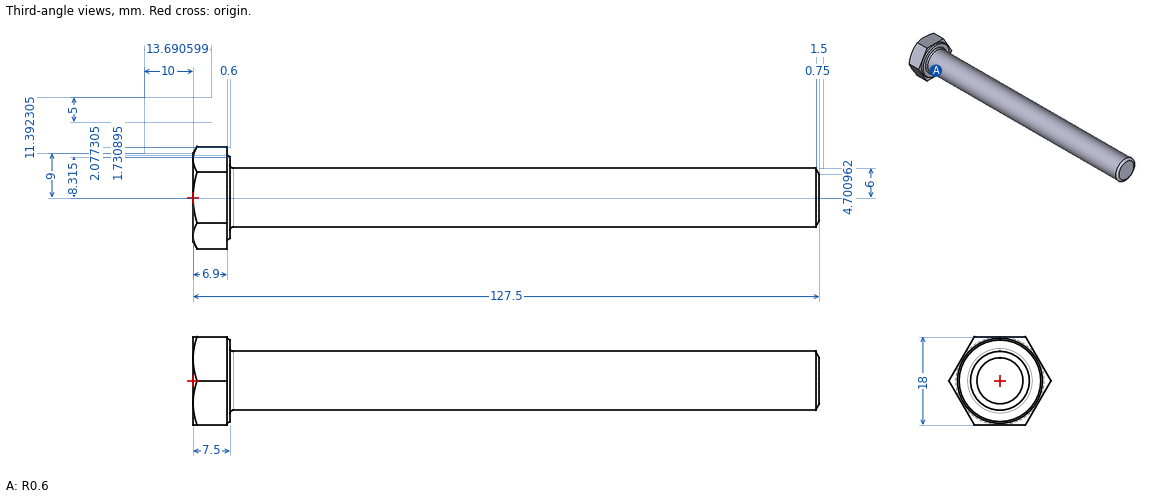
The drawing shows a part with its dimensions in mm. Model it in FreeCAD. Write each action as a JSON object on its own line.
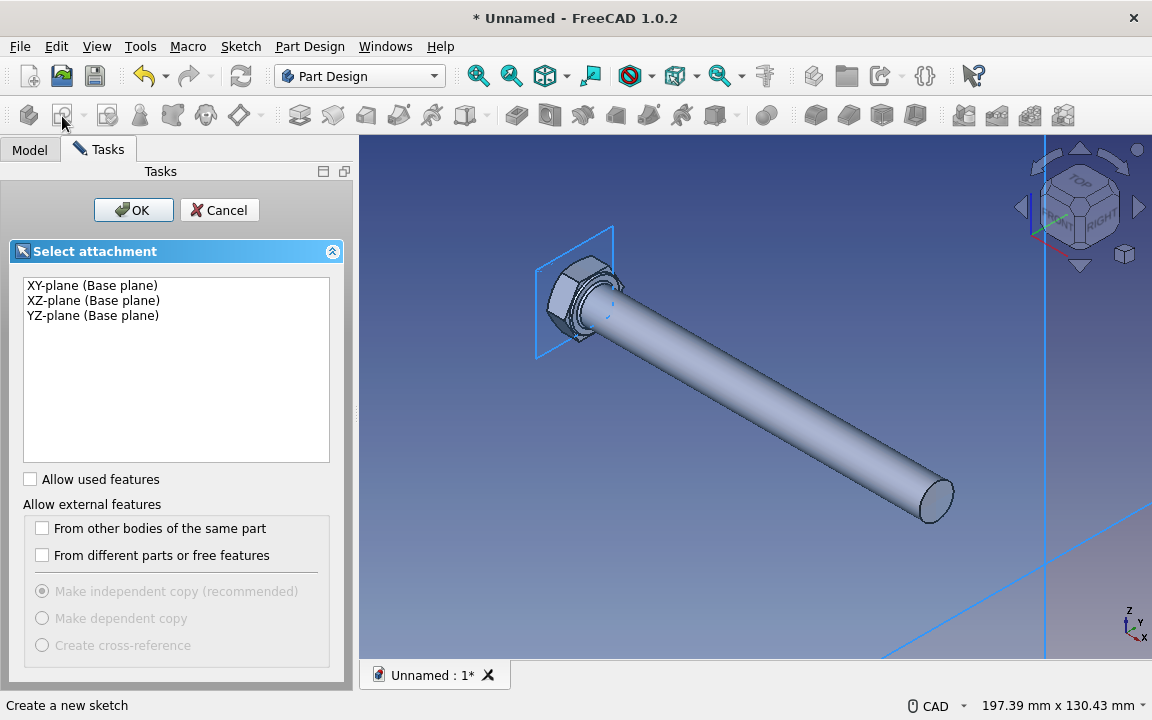
{"action": "left_click", "coordinate": [84, 286]}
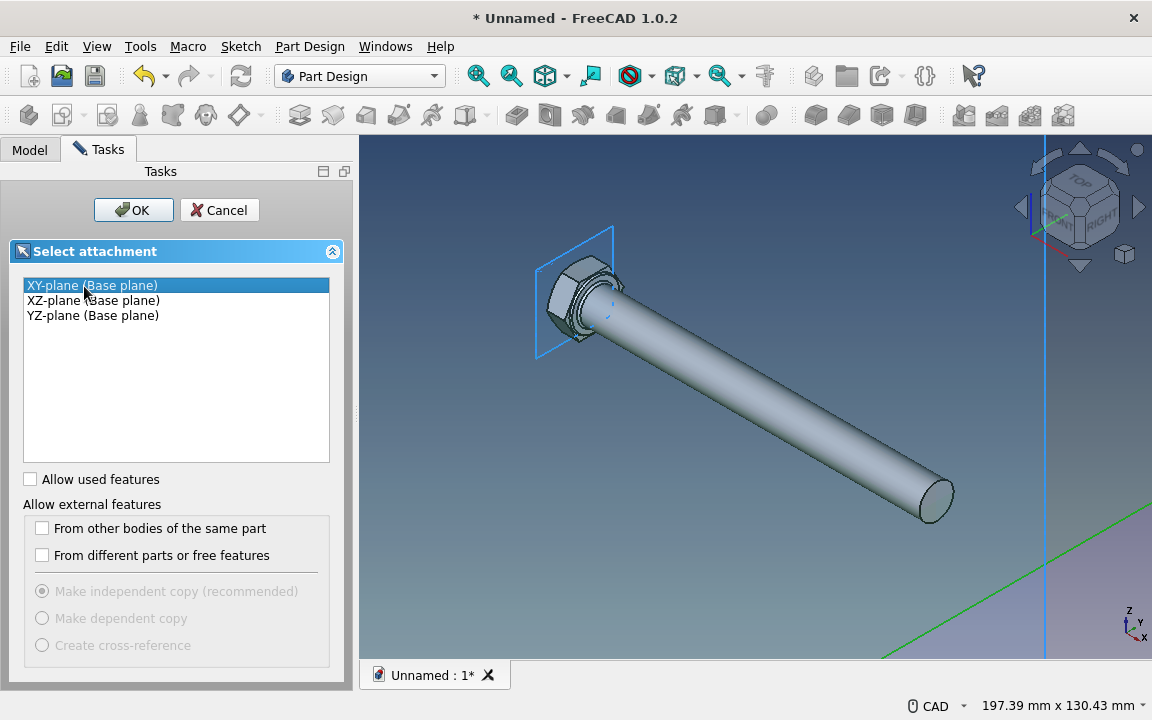
{"action": "left_click", "coordinate": [134, 210]}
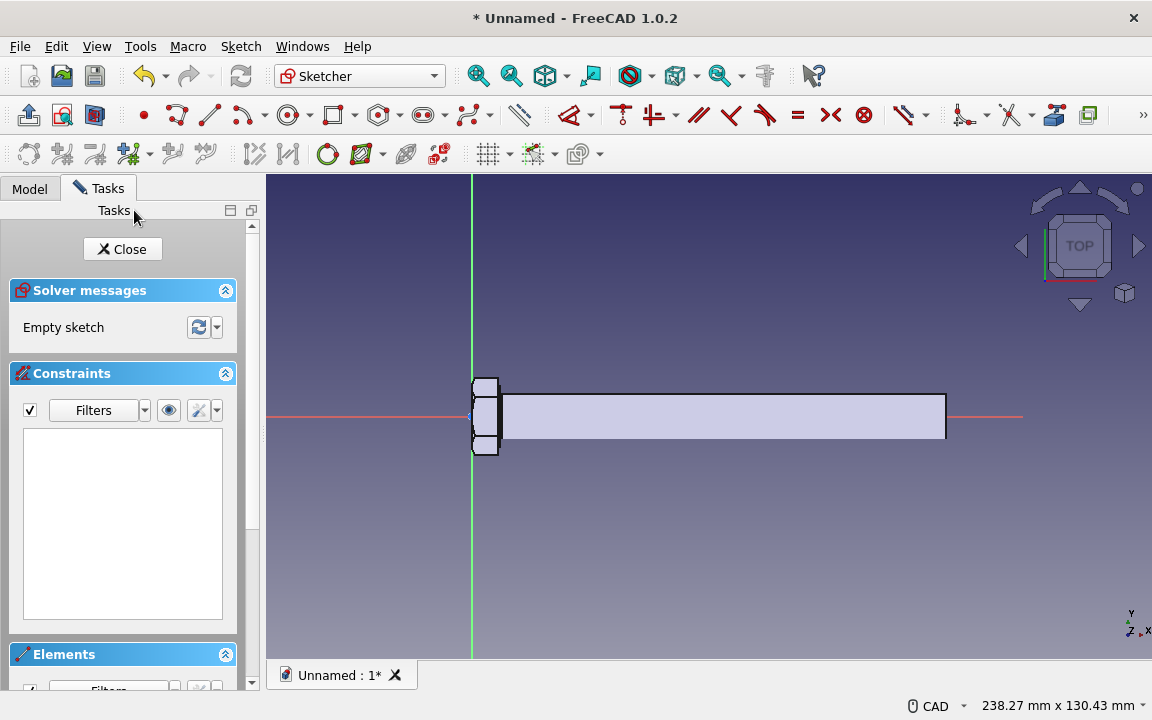
{"action": "left_click", "coordinate": [95, 116]}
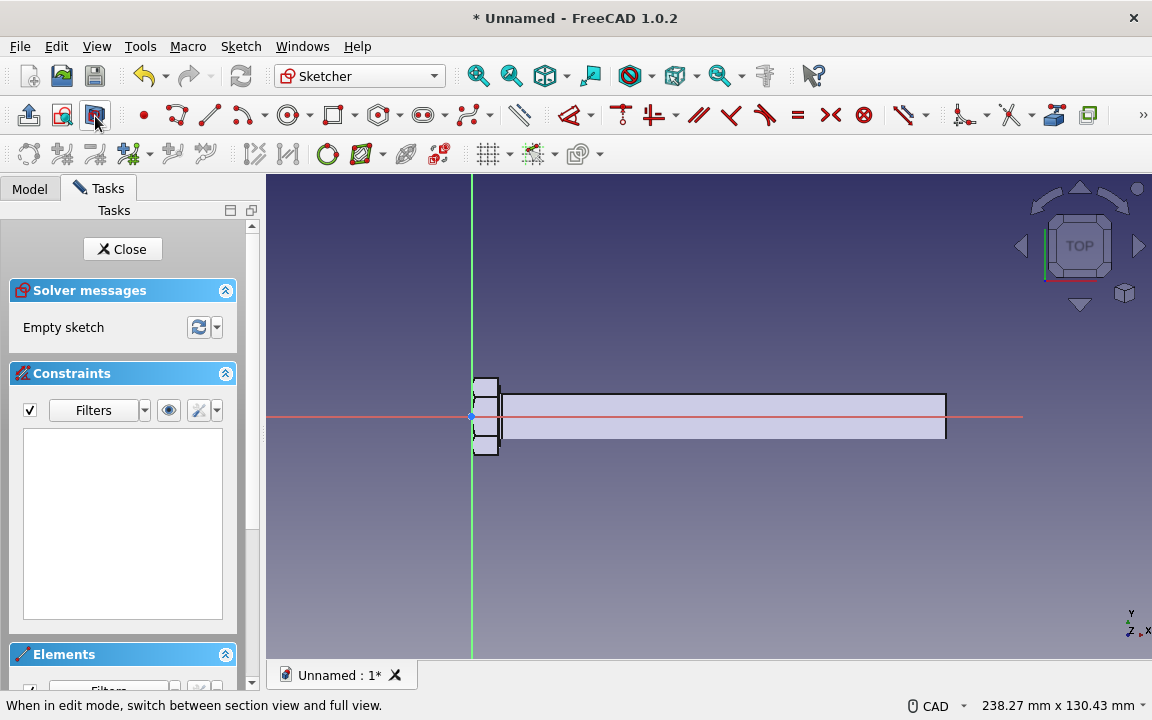
{"action": "scroll", "coordinate": [962, 396], "scroll_direction": "up", "scroll_amount": 15}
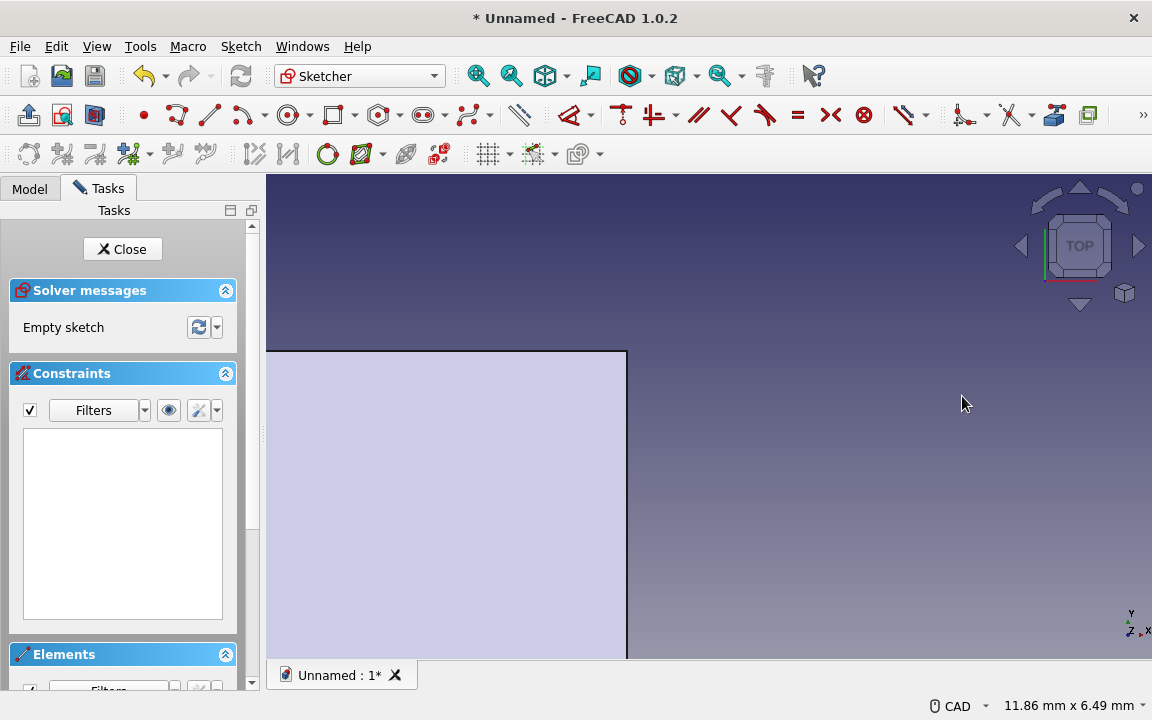
{"action": "scroll", "coordinate": [621, 392], "scroll_direction": "up", "scroll_amount": 6}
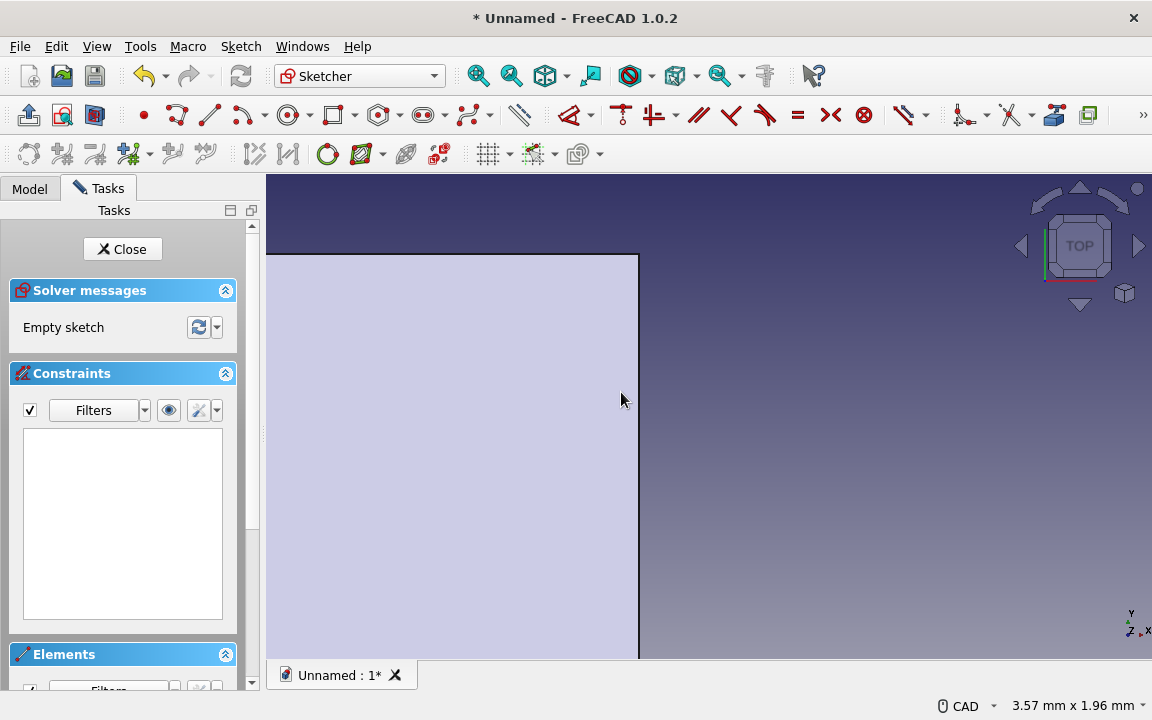
{"action": "left_click", "coordinate": [177, 116]}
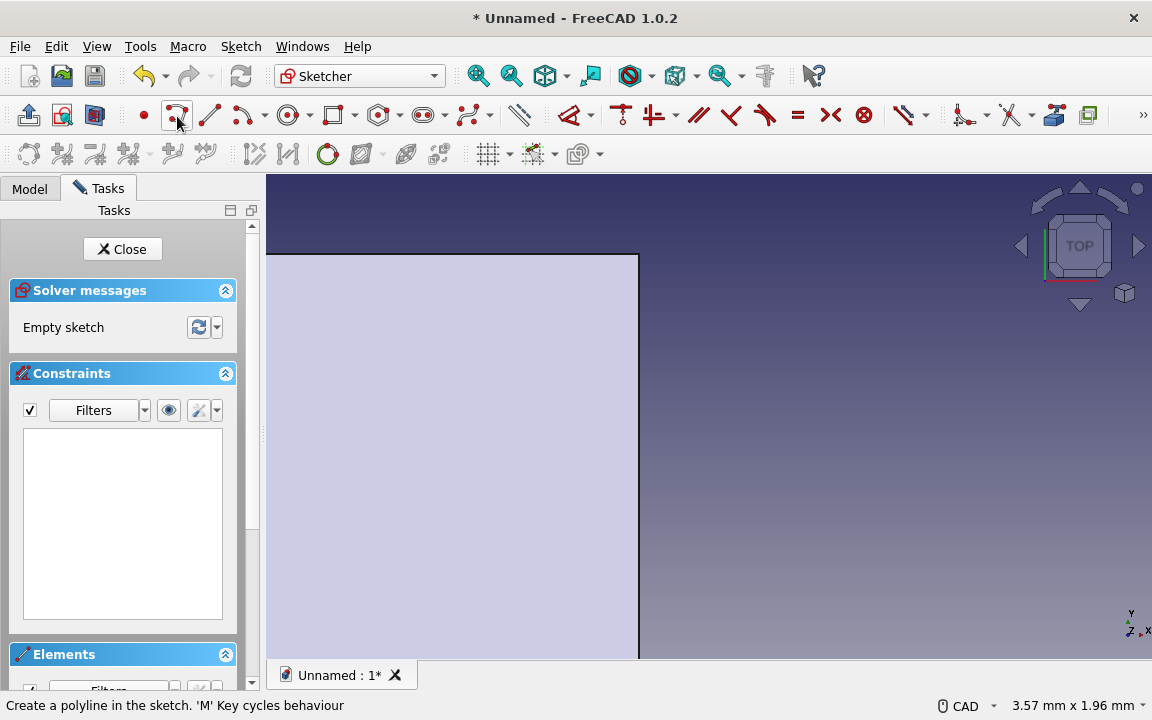
{"action": "left_click", "coordinate": [453, 254]}
{"action": "left_click", "coordinate": [639, 577]}
{"action": "left_click", "coordinate": [825, 254]}
{"action": "left_click", "coordinate": [453, 255]}
{"action": "key", "text": "Escape"}
{"action": "key", "text": "Escape"}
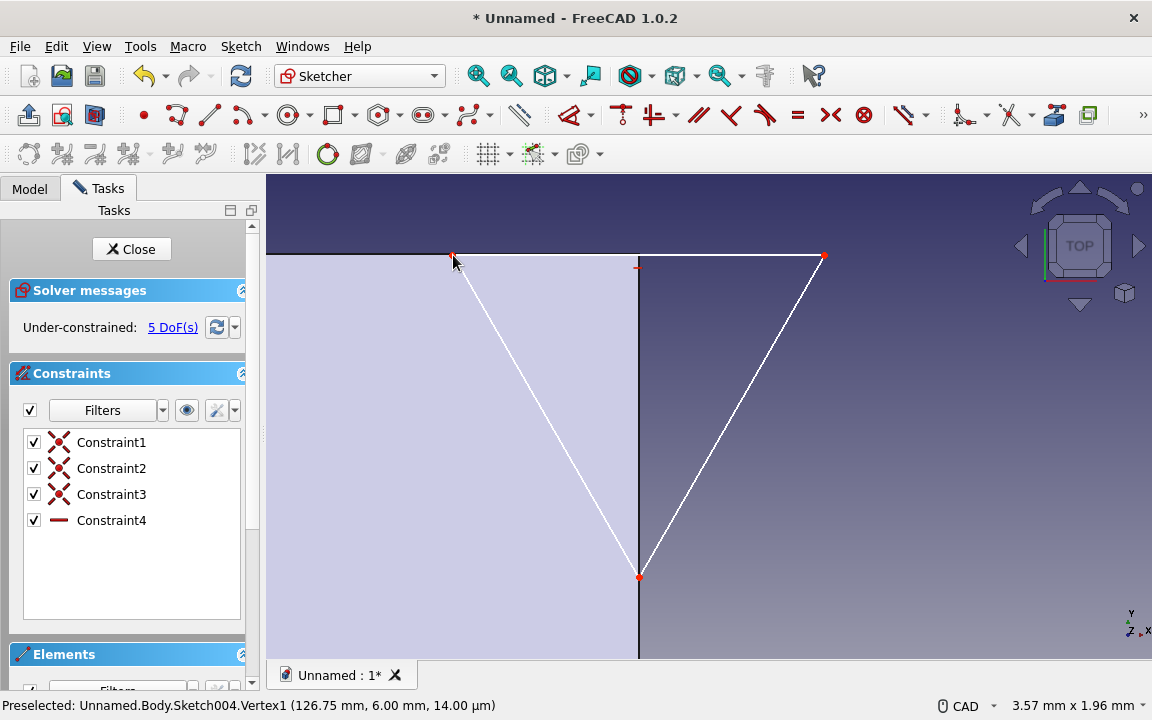
{"action": "left_click", "coordinate": [568, 116]}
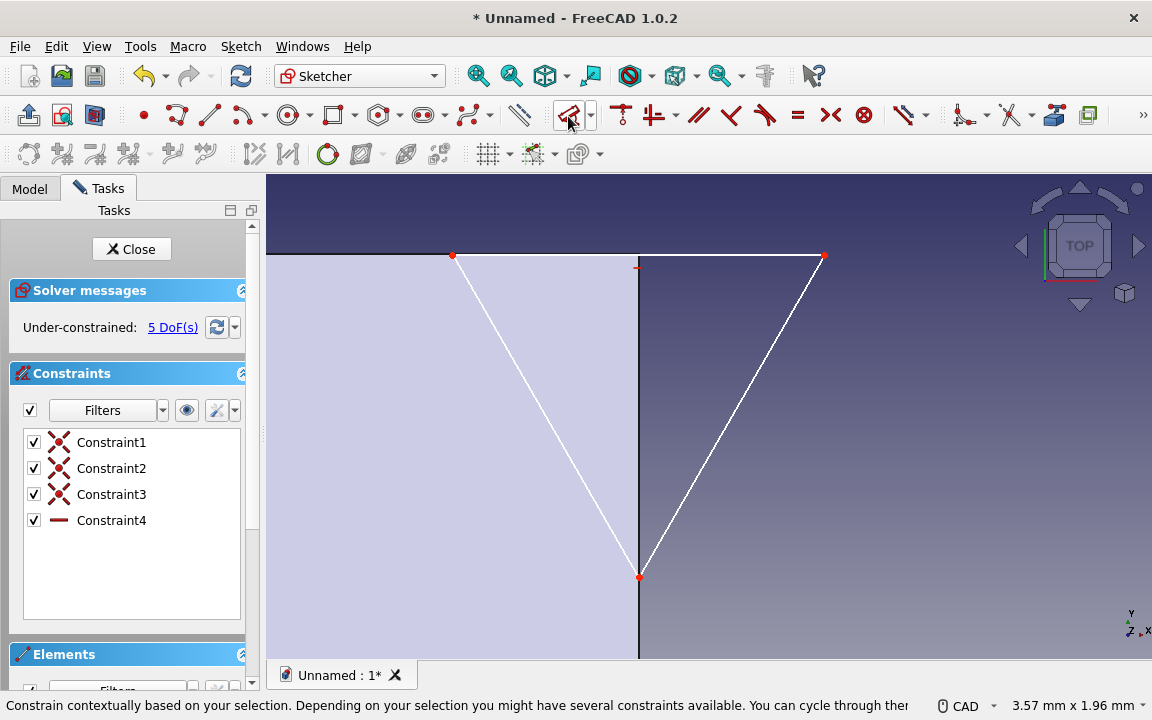
{"action": "left_click", "coordinate": [453, 255]}
{"action": "left_click", "coordinate": [487, 443]}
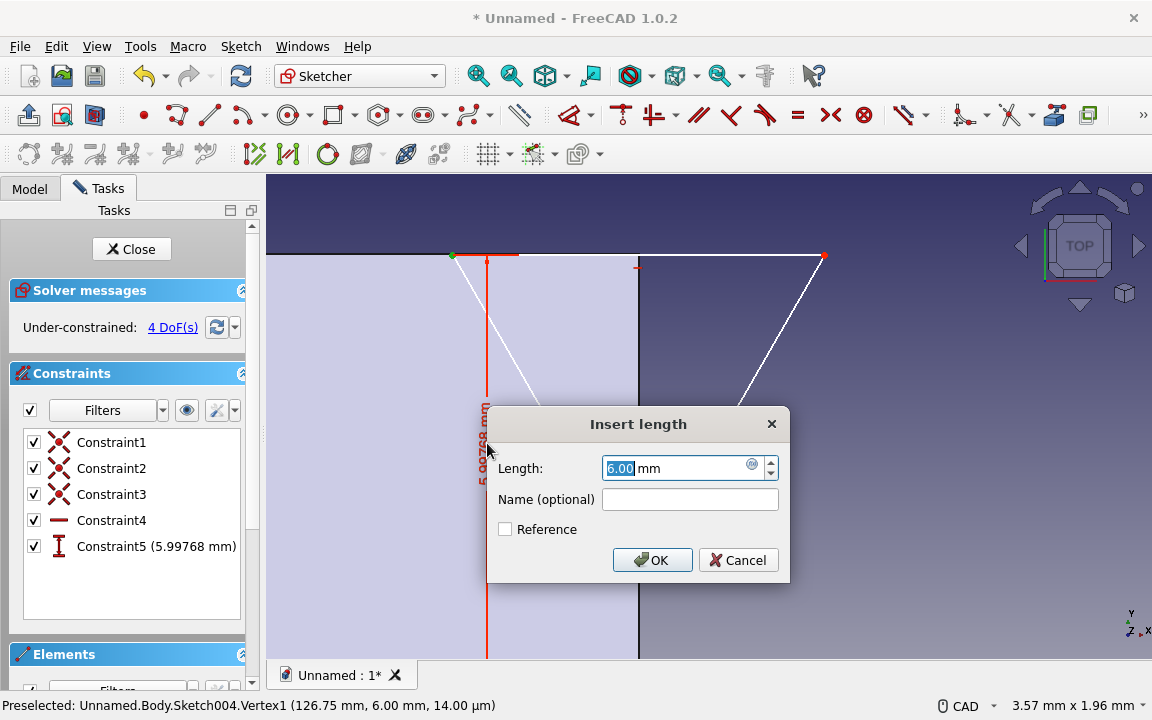
{"action": "type", "text": "6"}
{"action": "key", "text": "Return"}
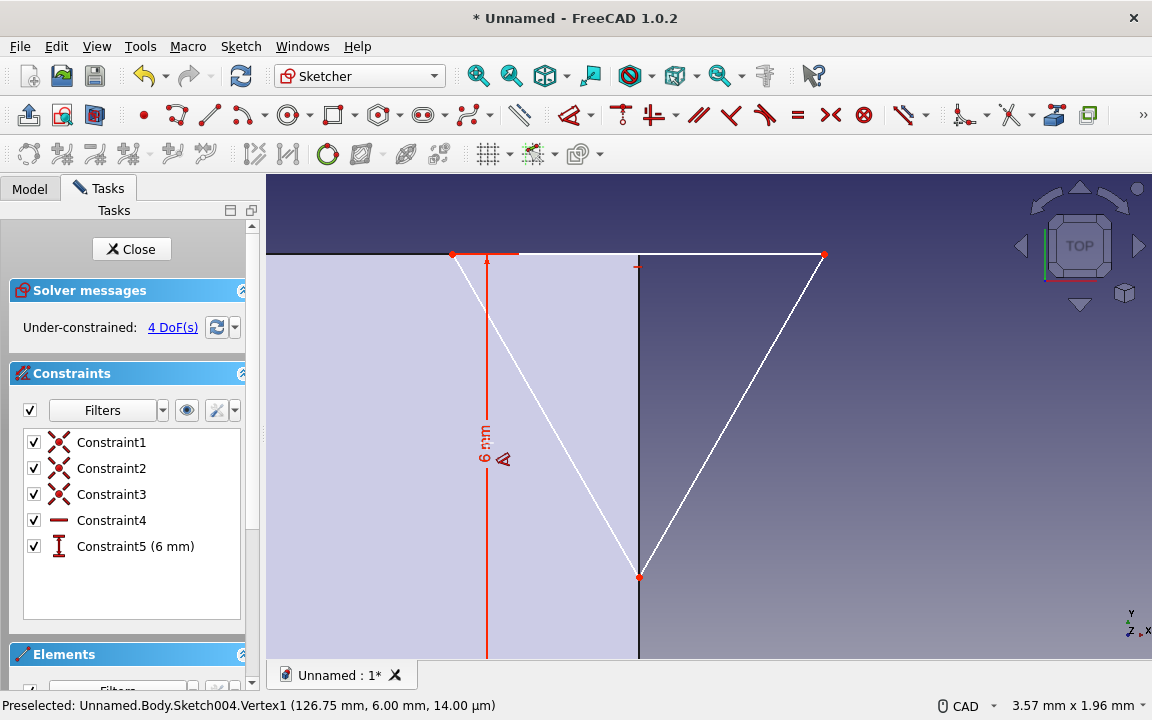
{"action": "left_click", "coordinate": [713, 254]}
{"action": "left_click", "coordinate": [639, 220]}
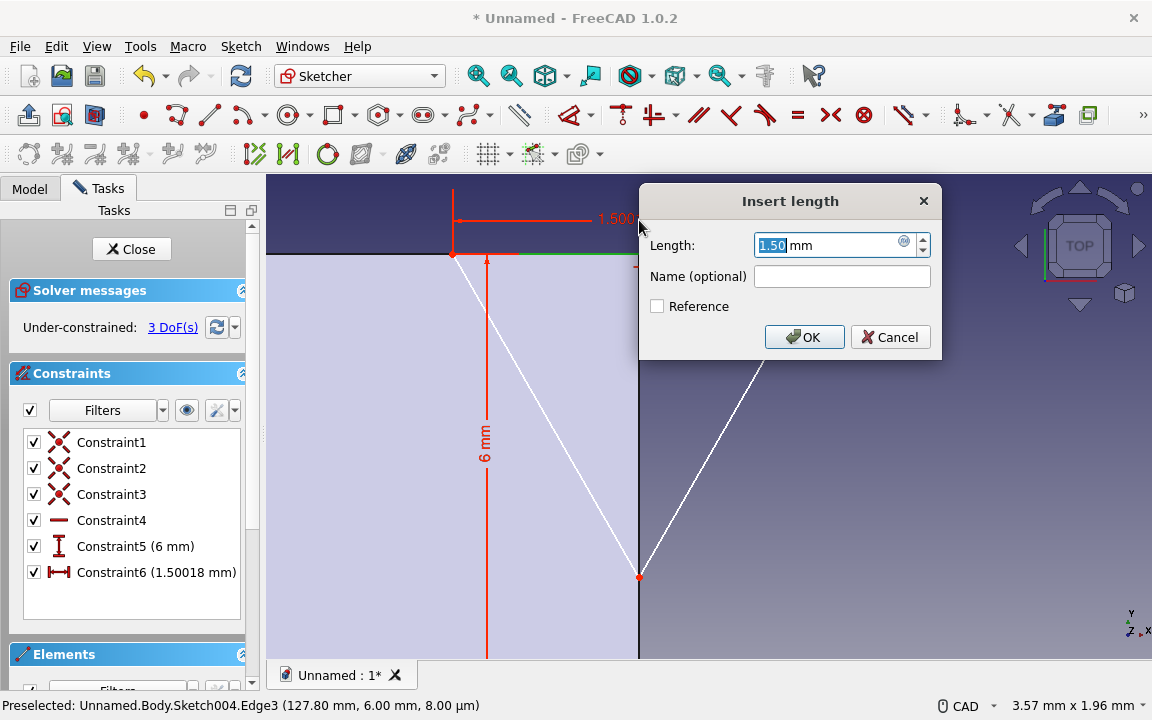
{"action": "type", "text": "1.5"}
{"action": "key", "text": "Return"}